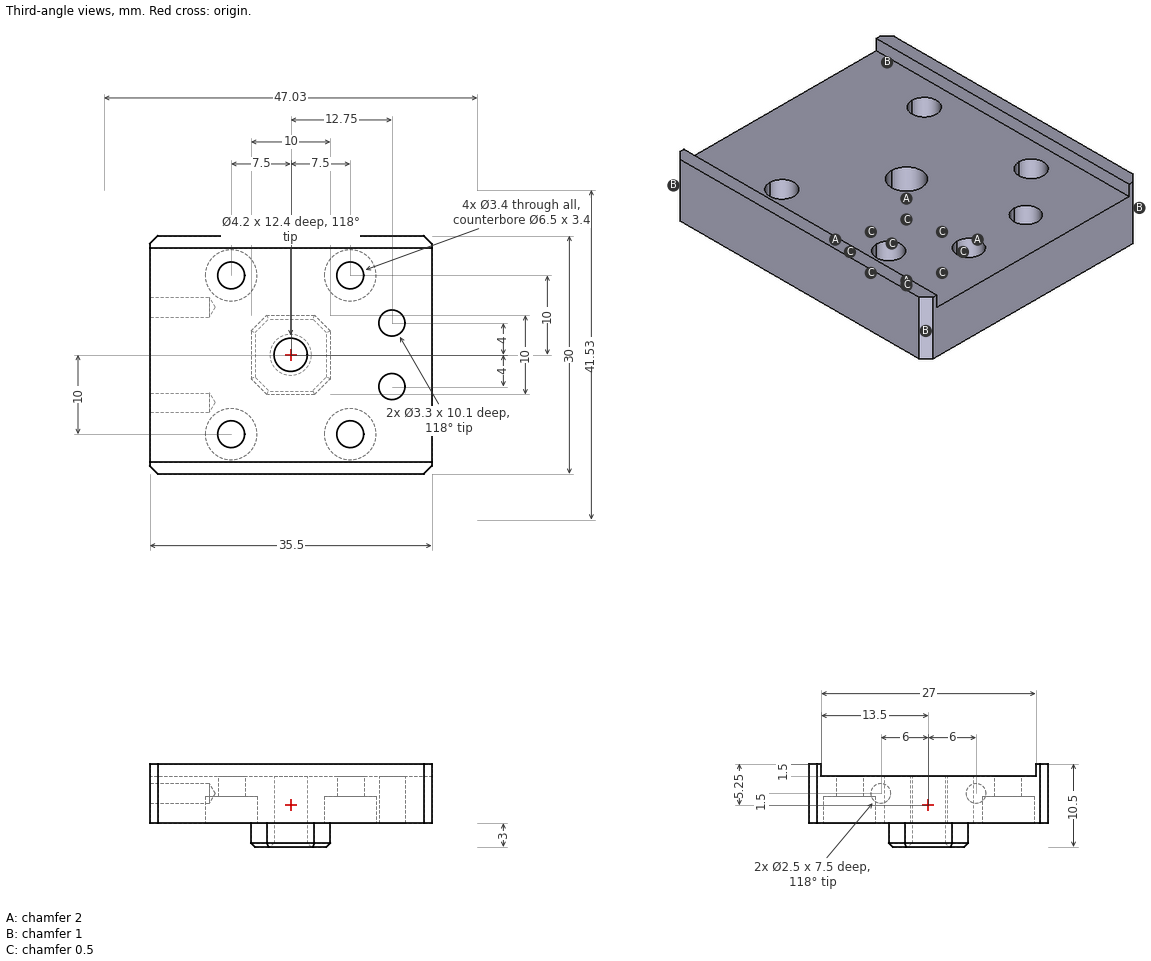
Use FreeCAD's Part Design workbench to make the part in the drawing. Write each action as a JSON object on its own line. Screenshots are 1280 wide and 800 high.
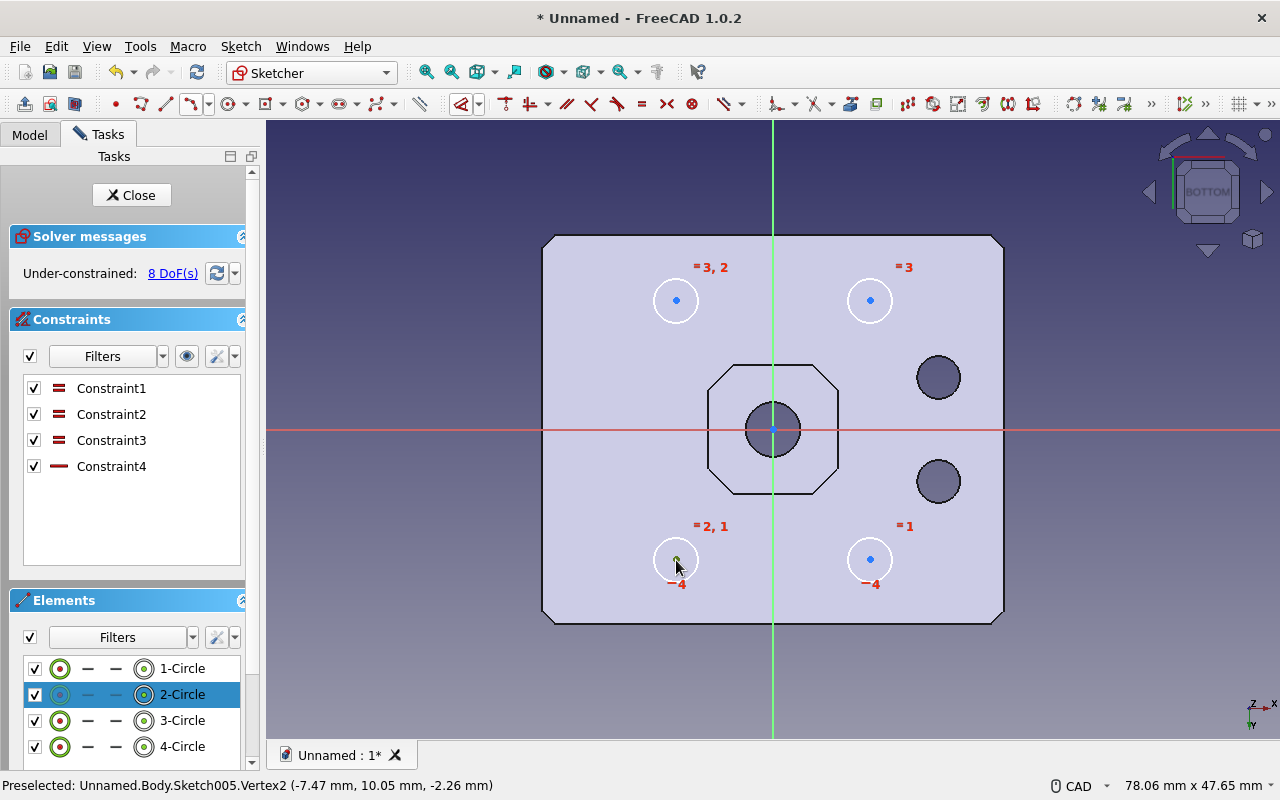
{"action": "left_click", "coordinate": [676, 301]}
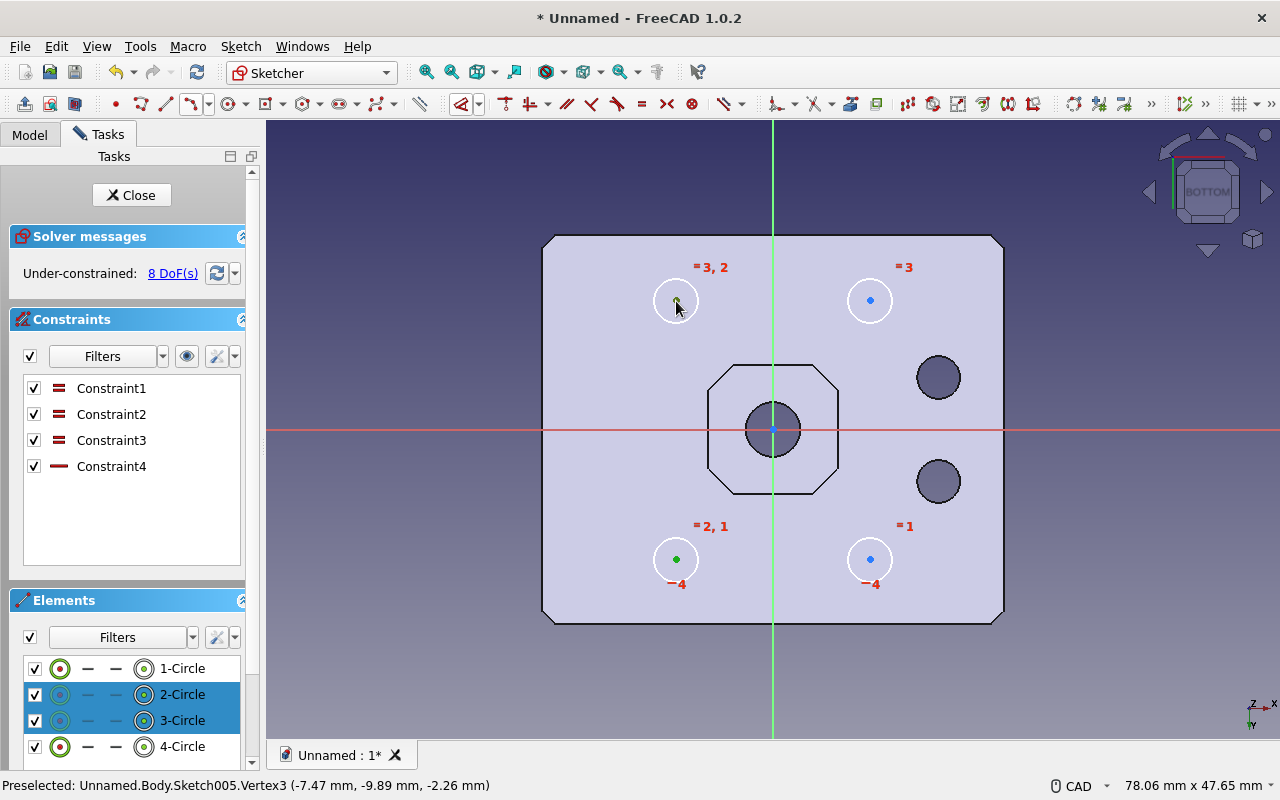
{"action": "key", "text": "v"}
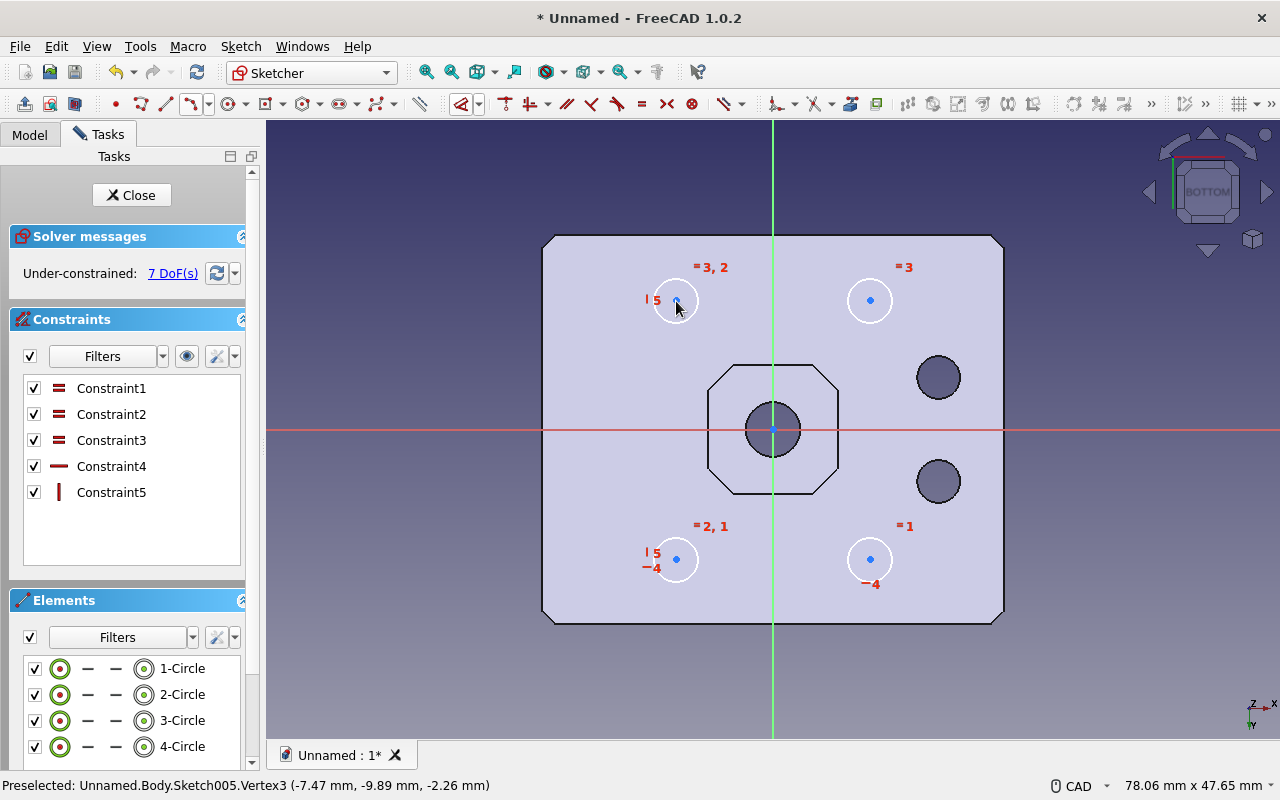
{"action": "left_click", "coordinate": [870, 560]}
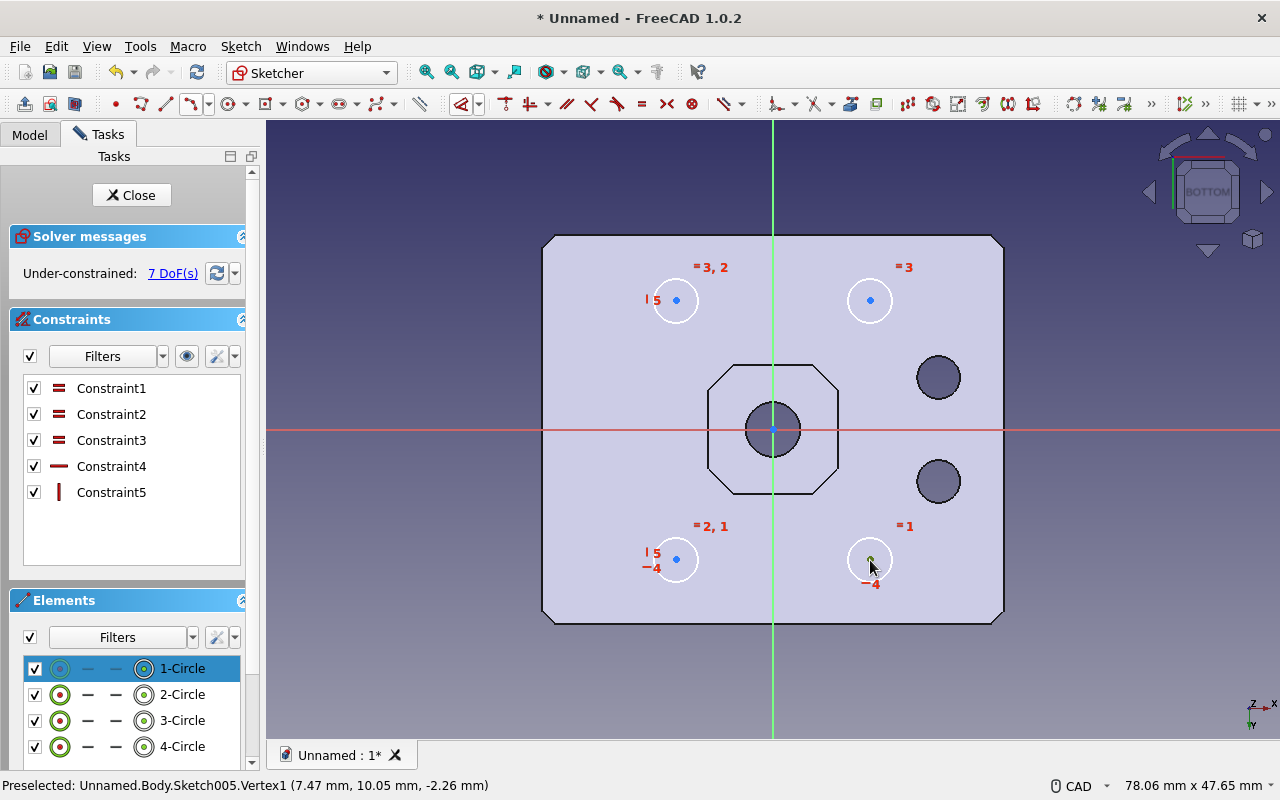
{"action": "left_click", "coordinate": [870, 301]}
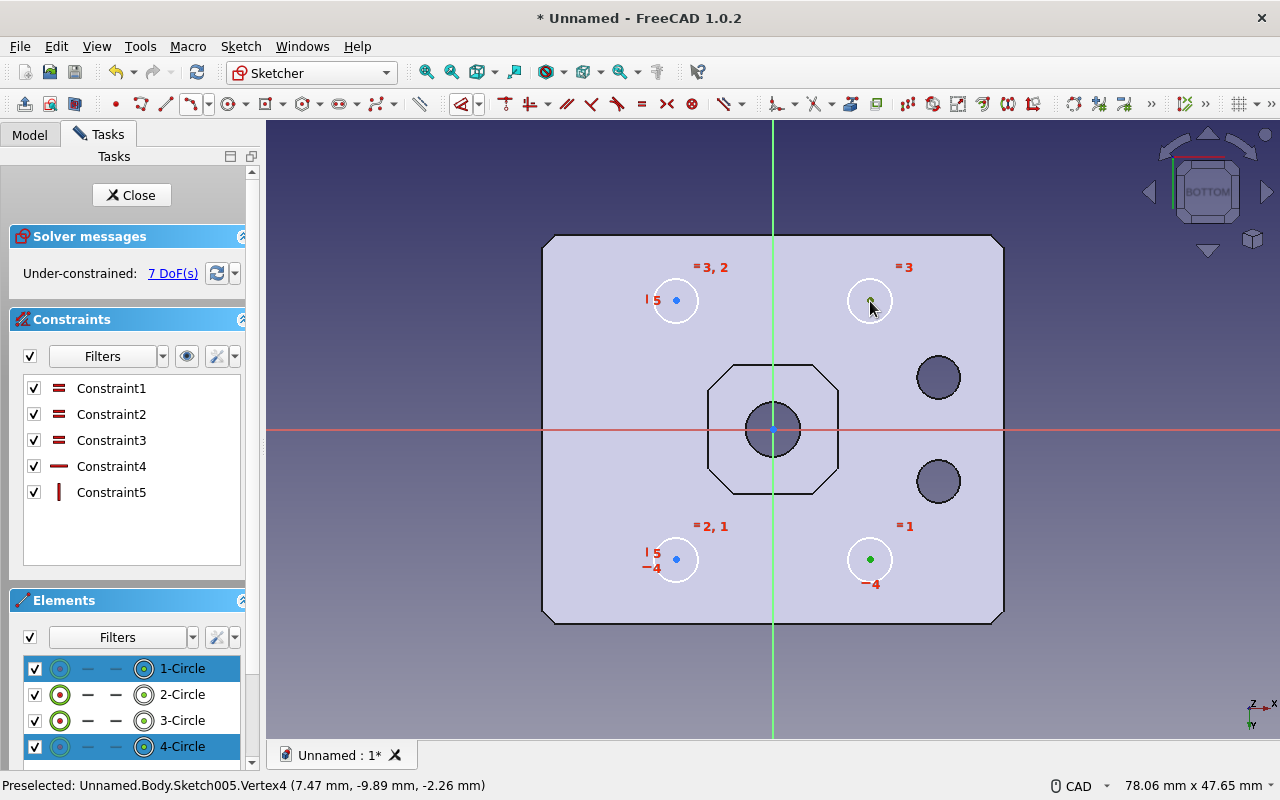
{"action": "key", "text": "v"}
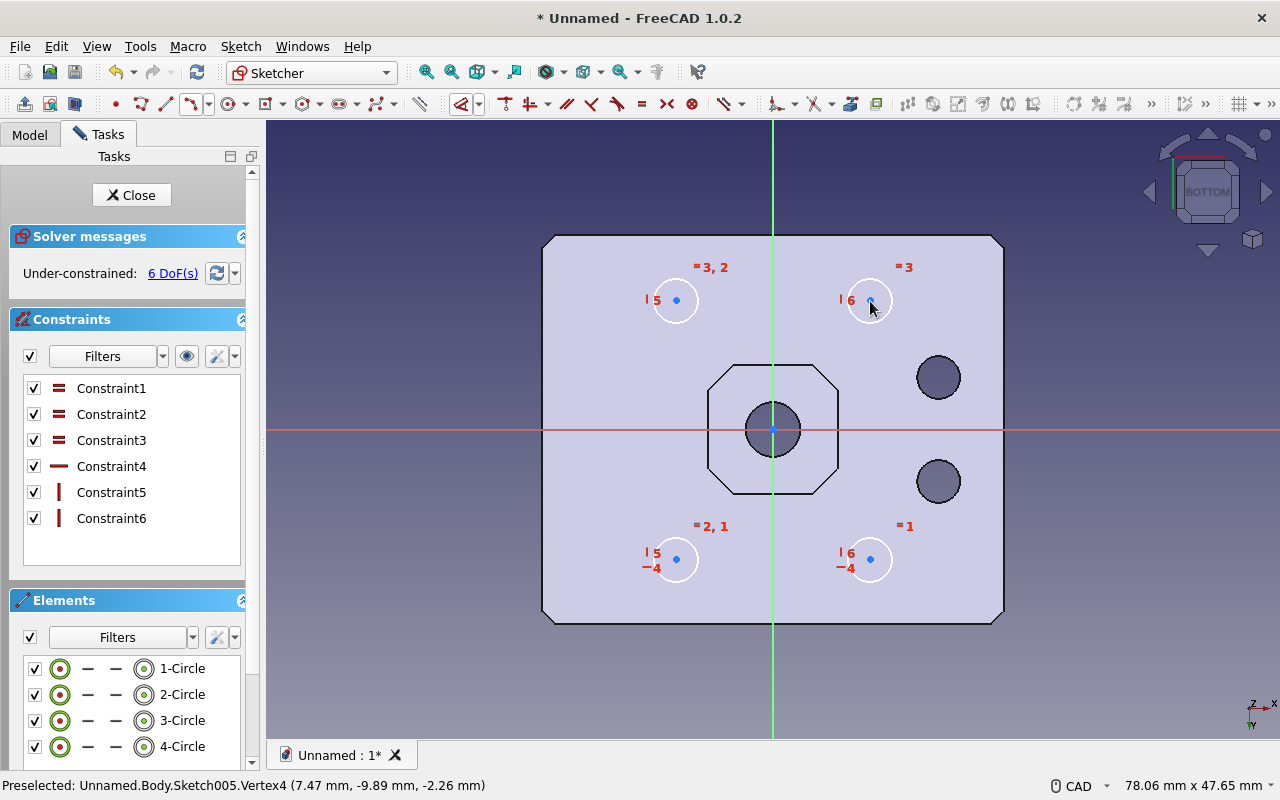
{"action": "left_click", "coordinate": [676, 301]}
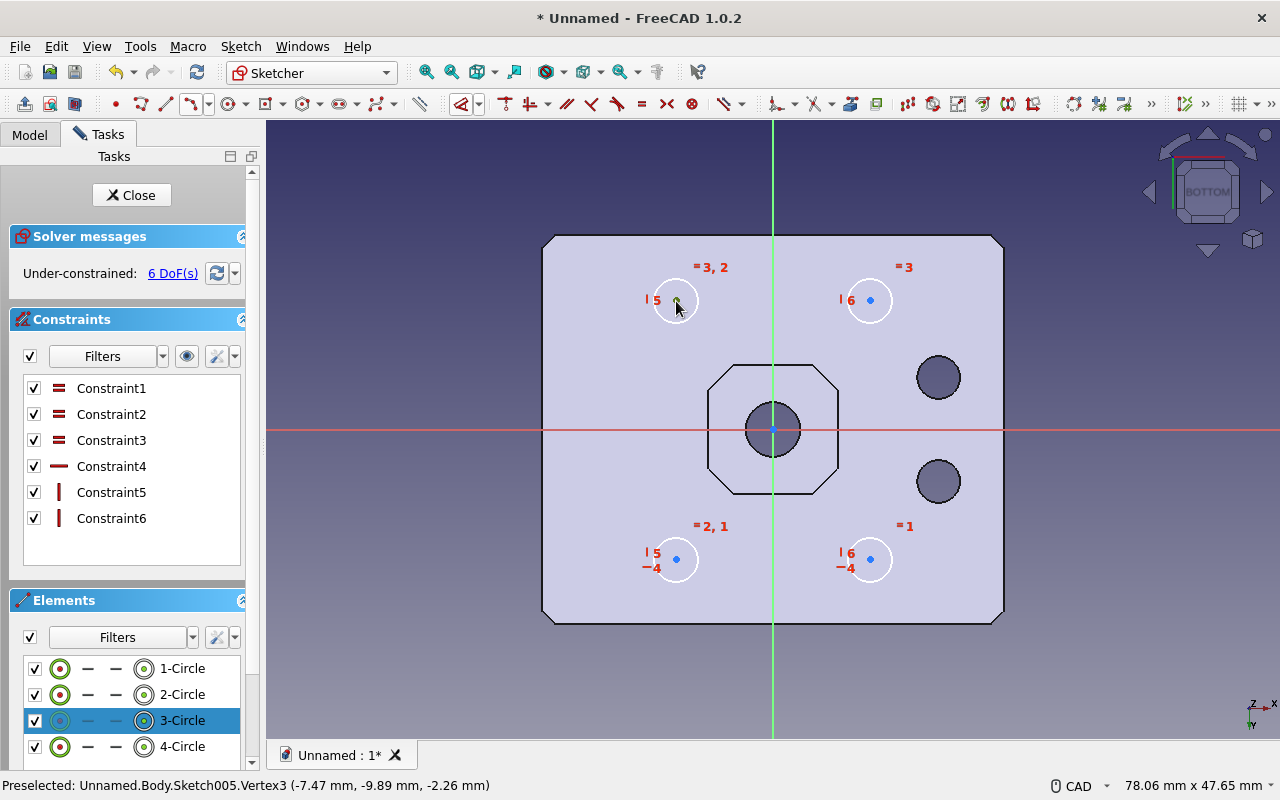
{"action": "left_click", "coordinate": [870, 301]}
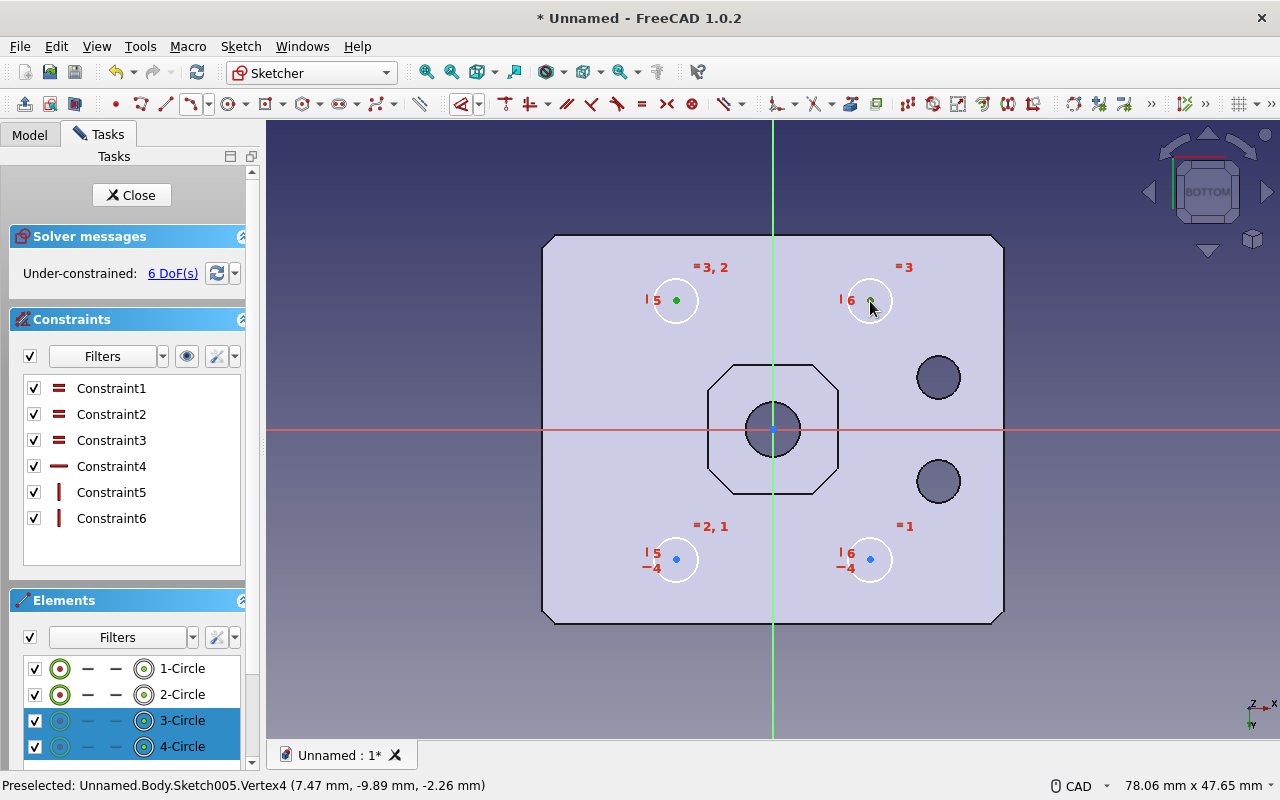
{"action": "key", "text": "h"}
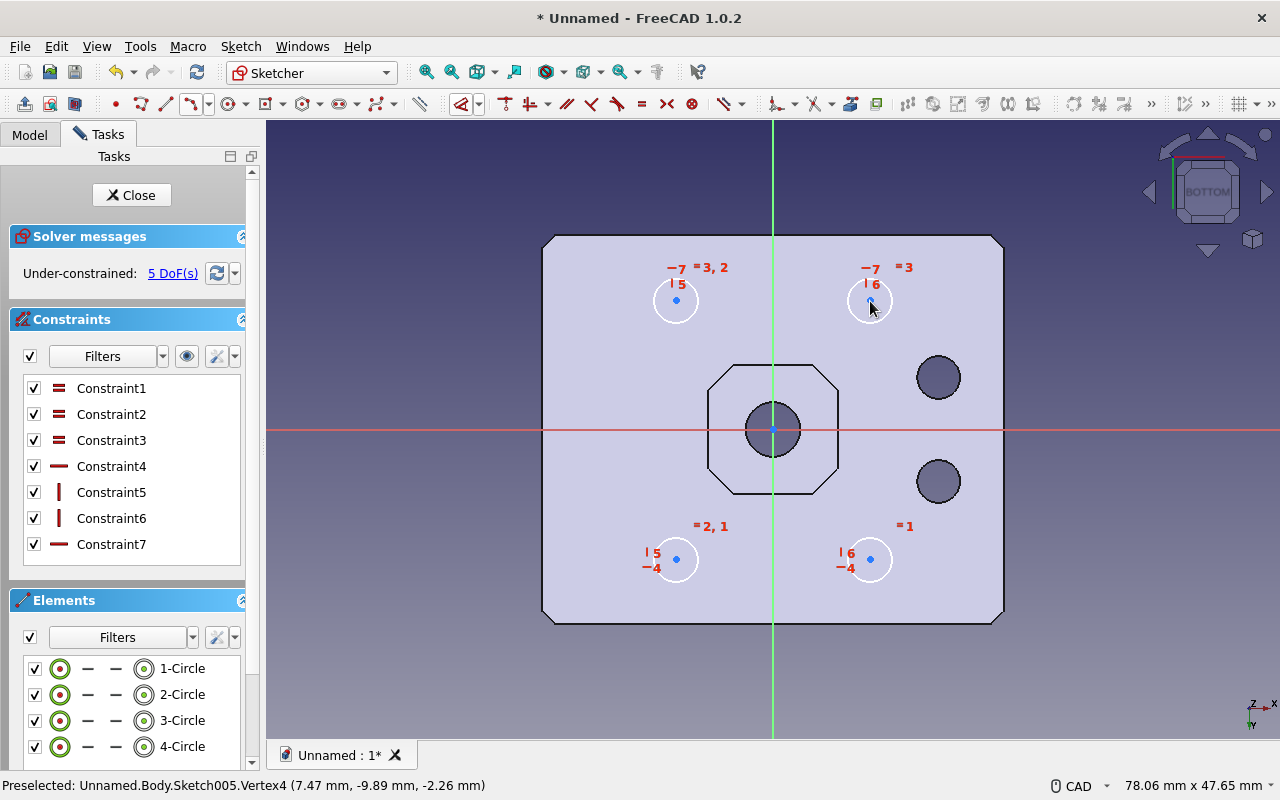
{"action": "key", "text": "d"}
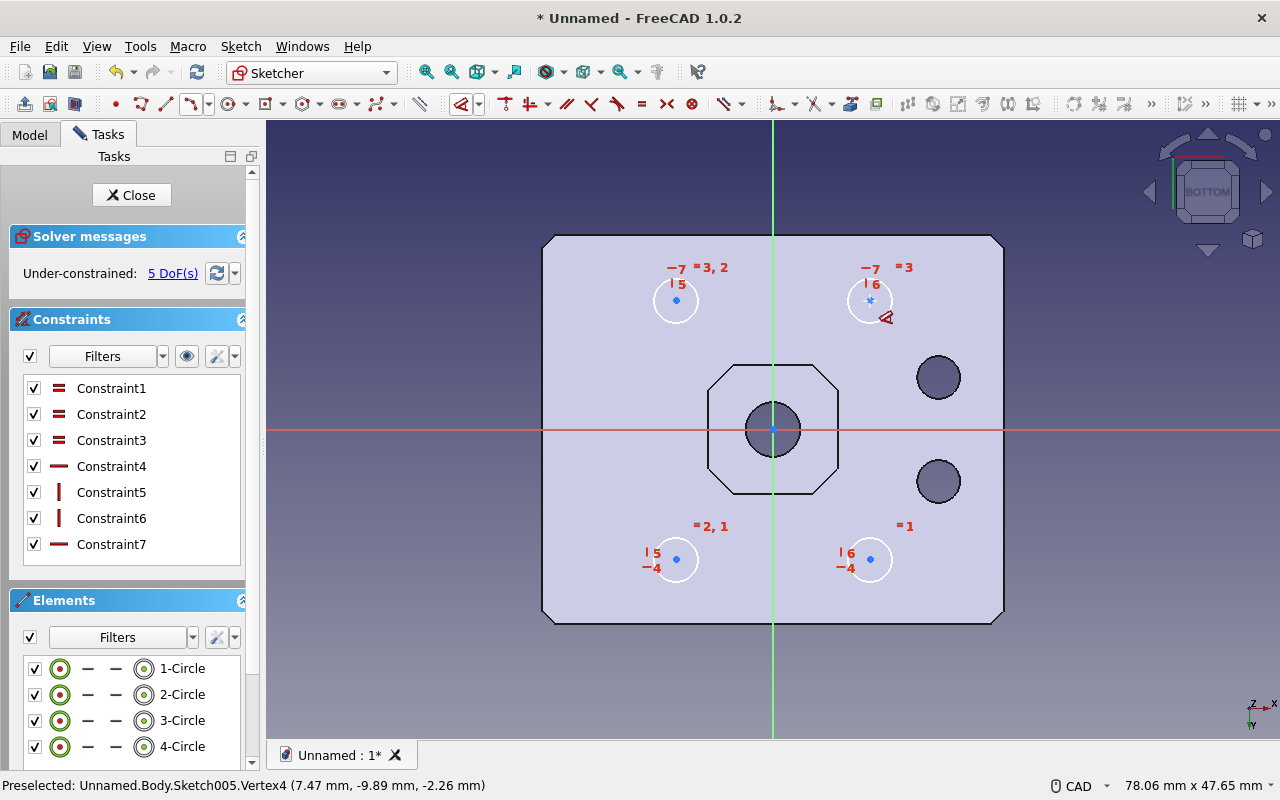
{"action": "left_click", "coordinate": [885, 544]}
{"action": "left_click", "coordinate": [907, 521]}